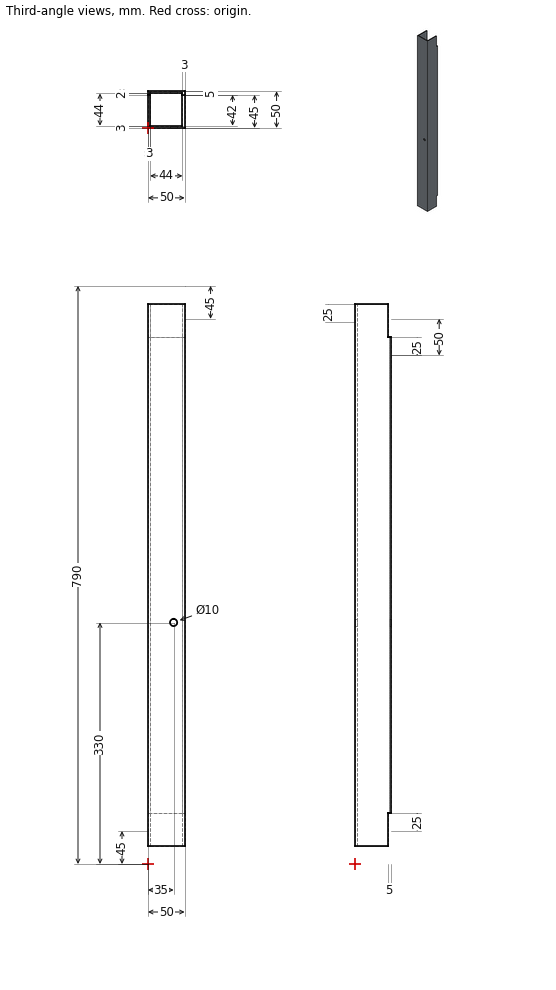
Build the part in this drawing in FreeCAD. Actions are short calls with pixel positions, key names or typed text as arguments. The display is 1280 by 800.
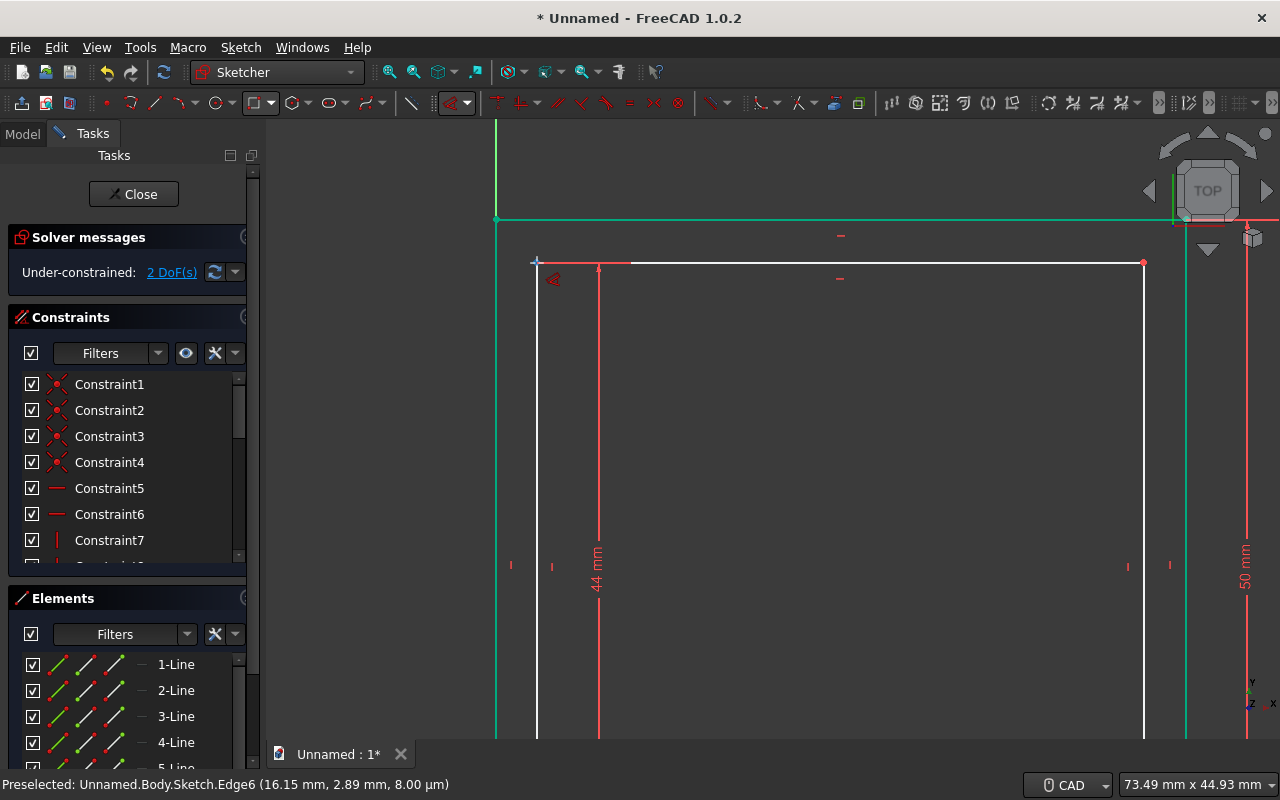
click(537, 263)
click(517, 205)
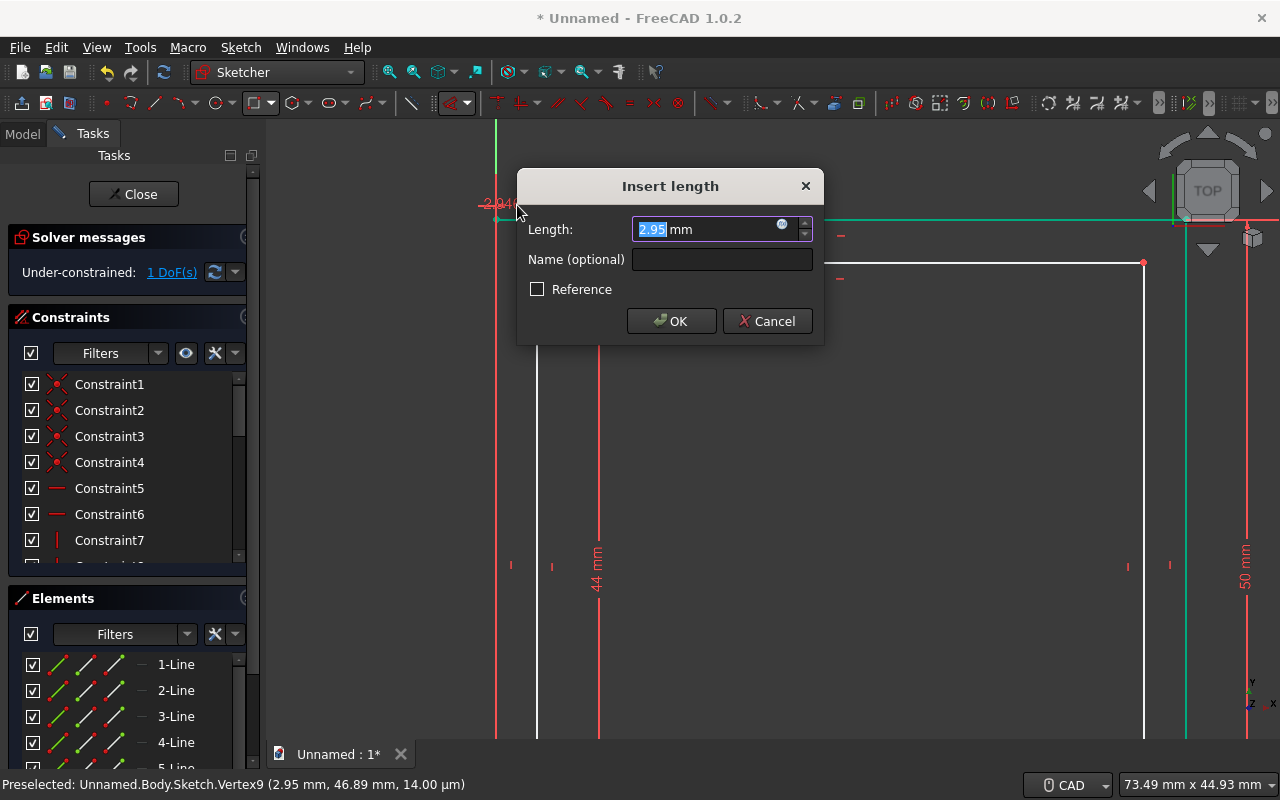
text(3)
key(Return)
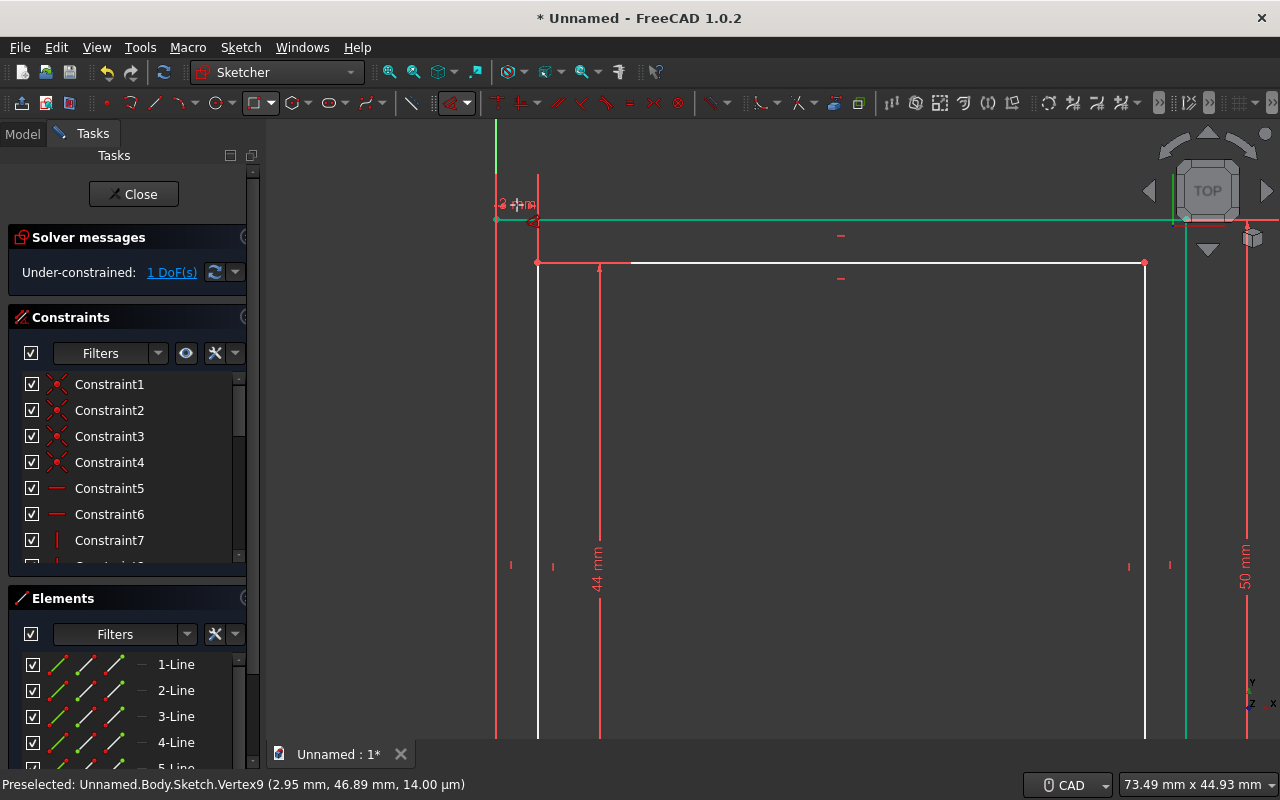
scroll(538, 264, down, 3)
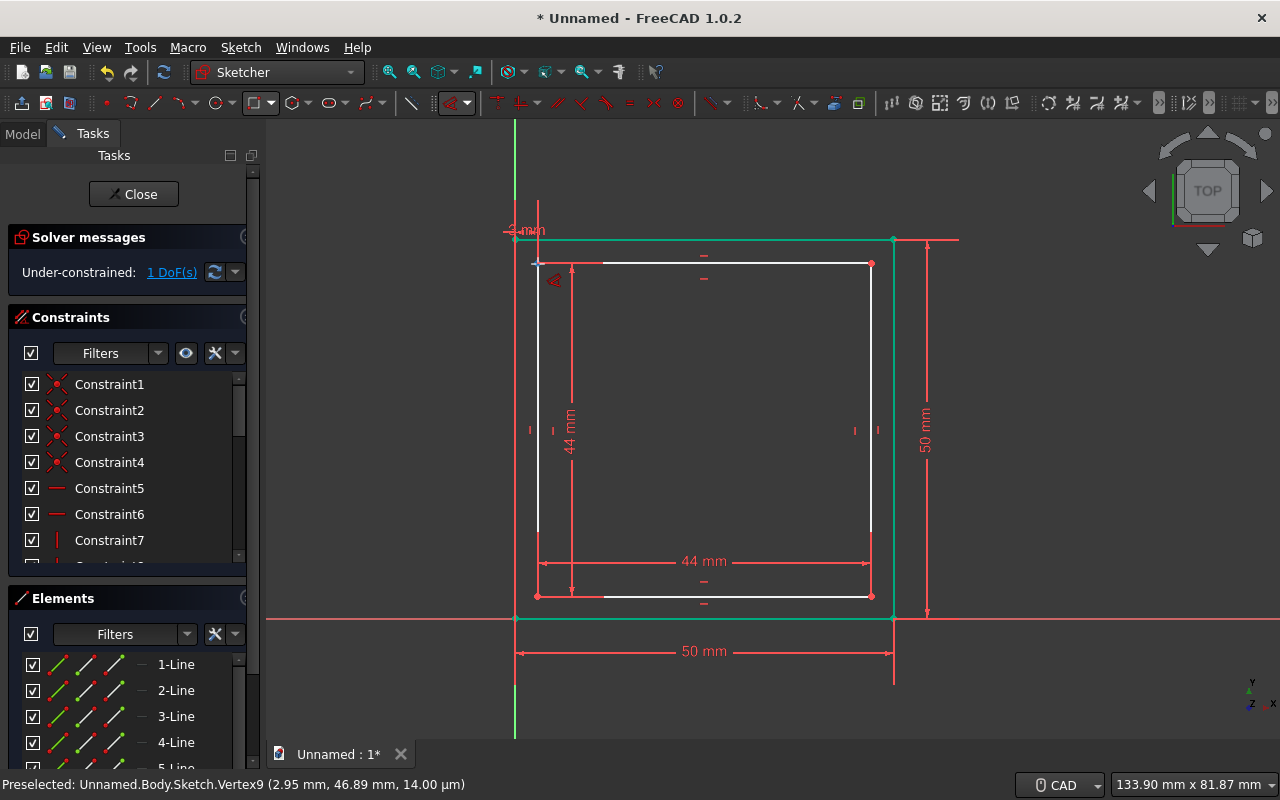
scroll(538, 597, up, 3)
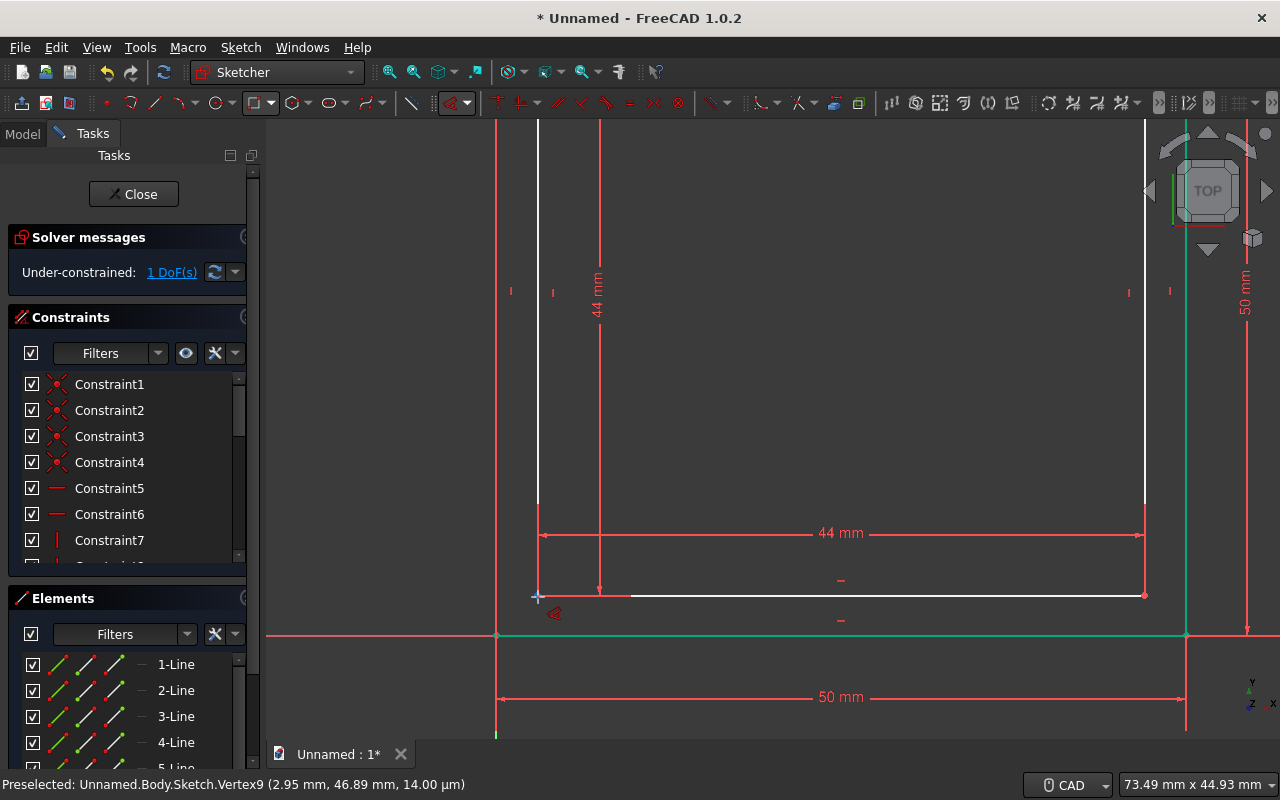
click(538, 596)
click(462, 616)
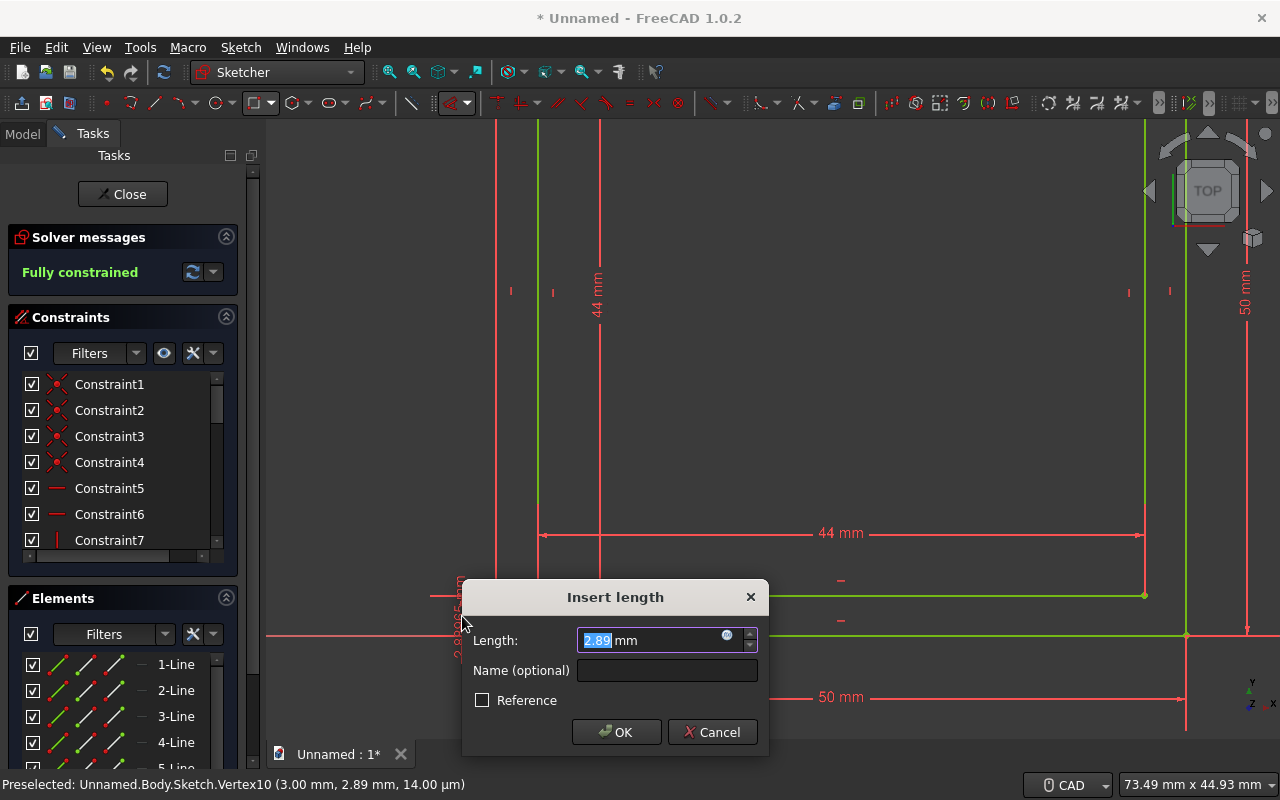
text(3)
key(Return)
key(Escape)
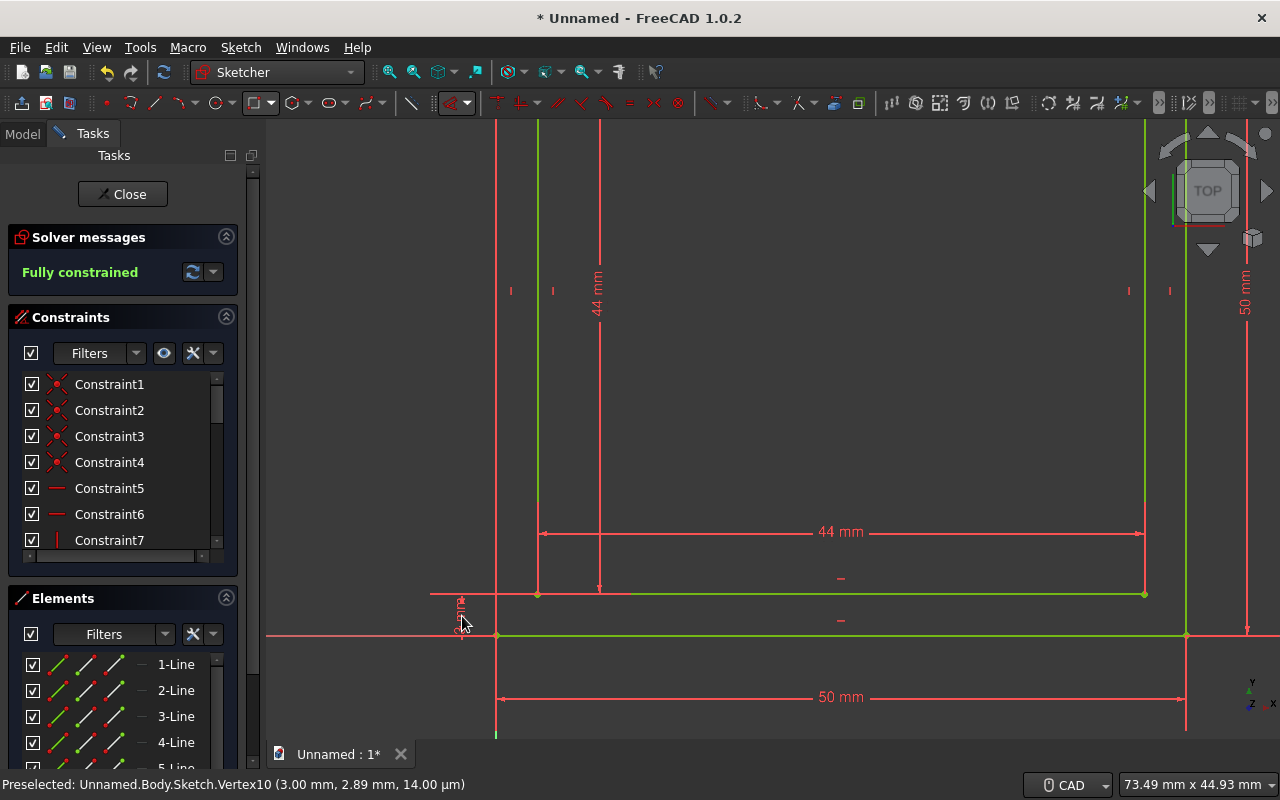
click(123, 194)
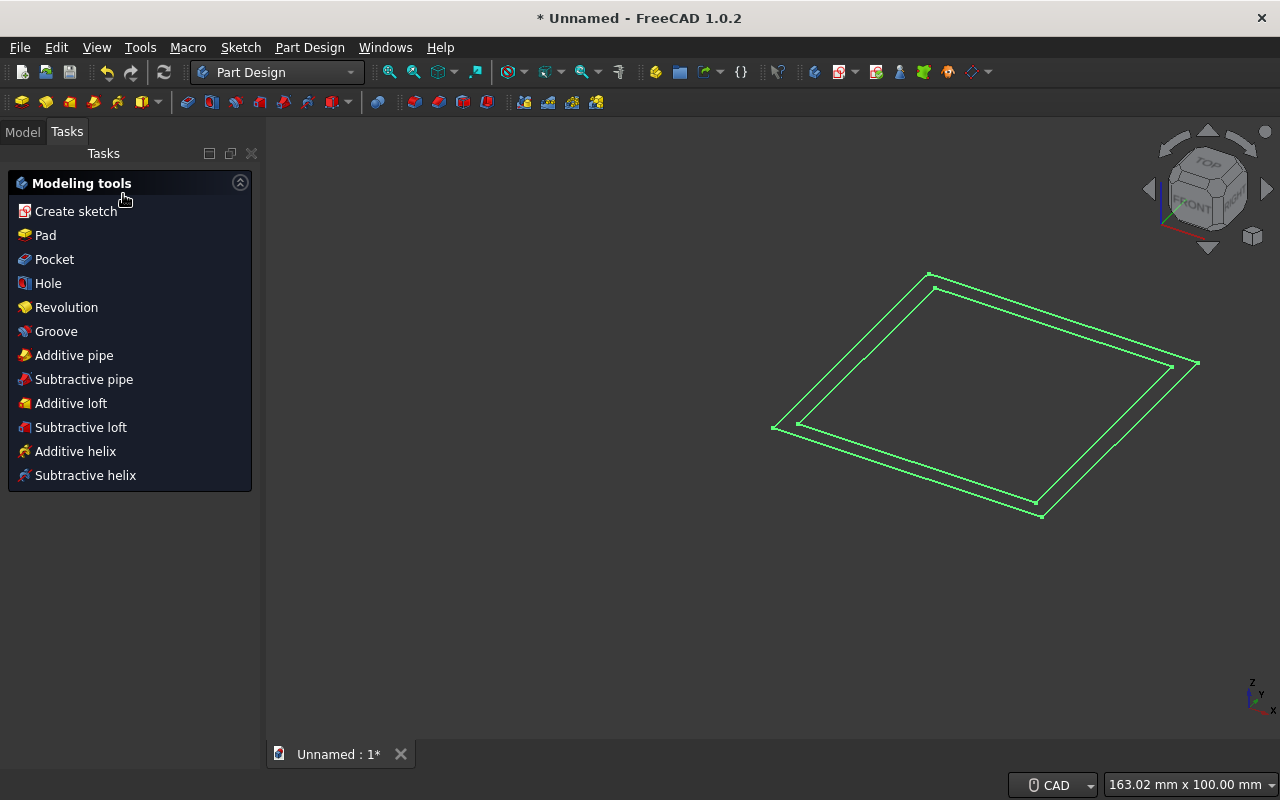
click(22, 102)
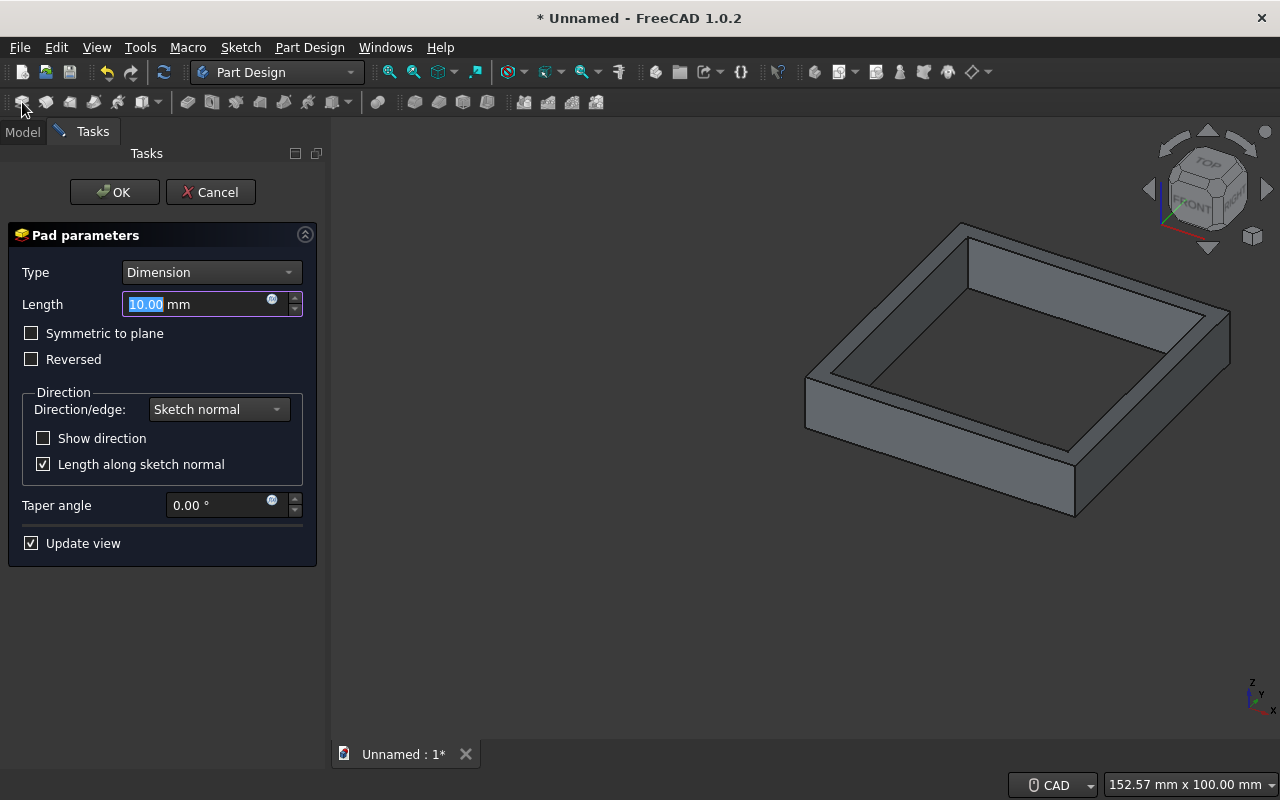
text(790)
key(Tab)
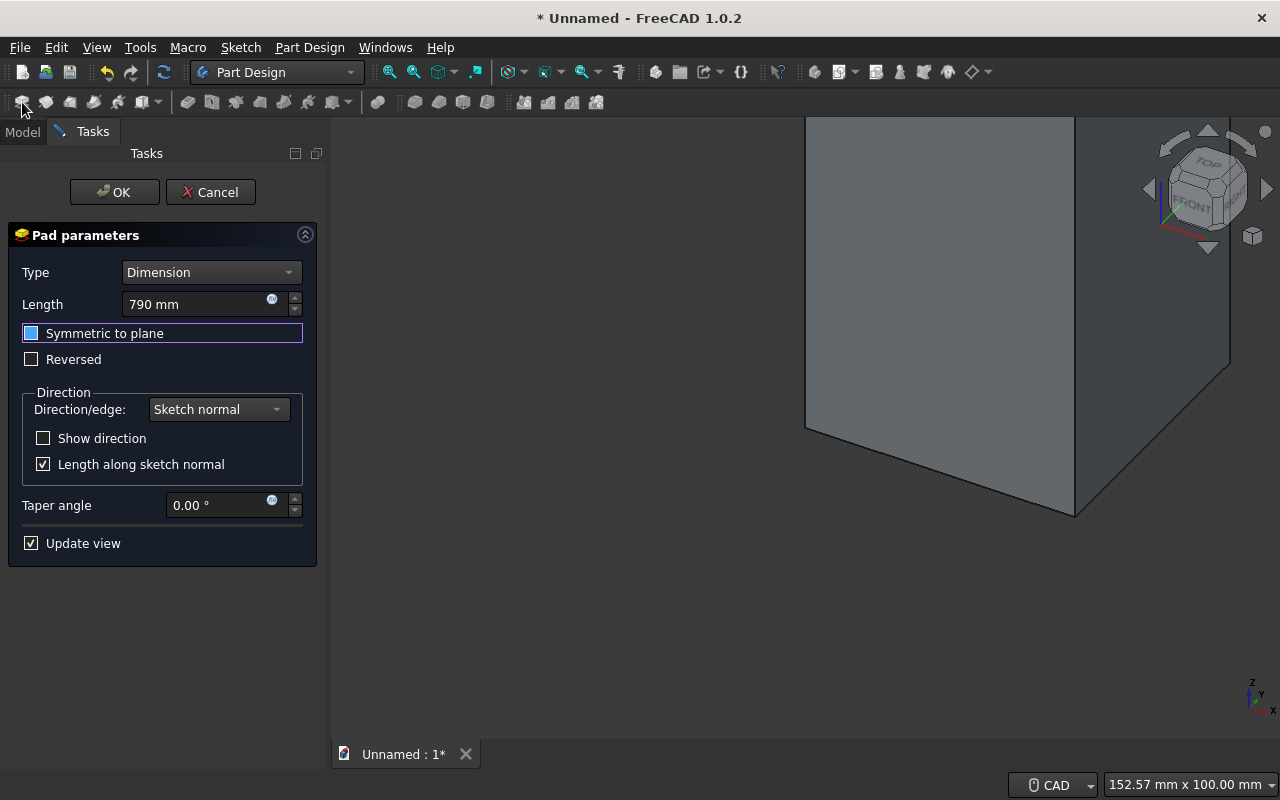
click(115, 192)